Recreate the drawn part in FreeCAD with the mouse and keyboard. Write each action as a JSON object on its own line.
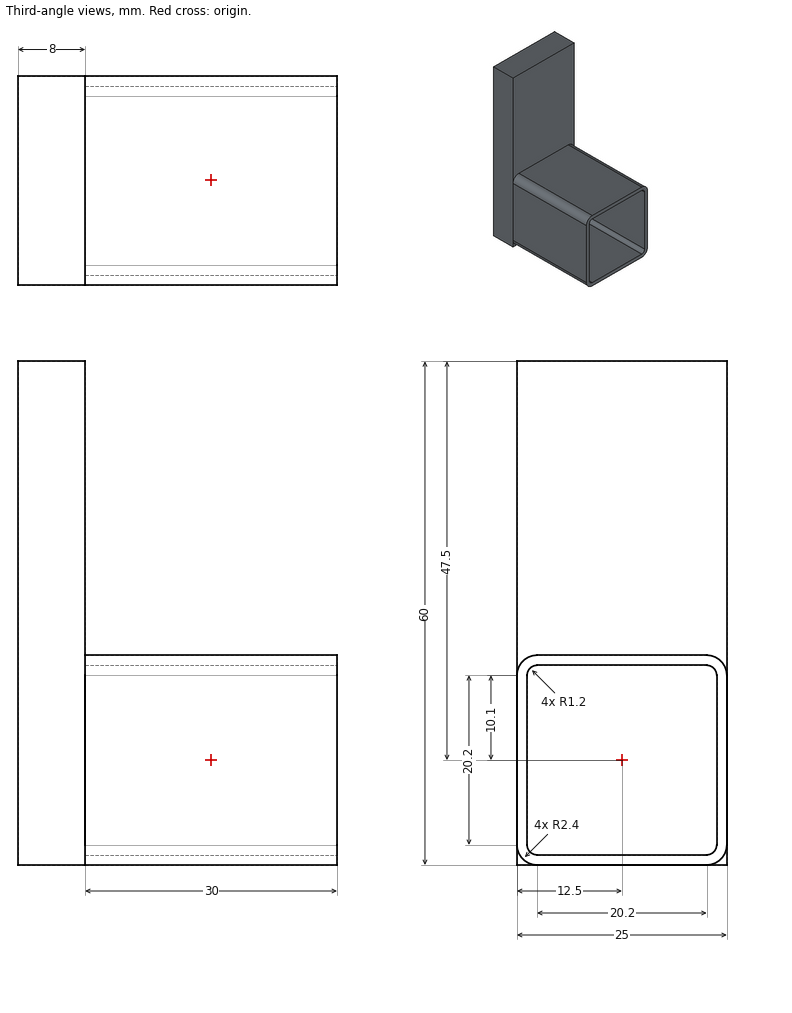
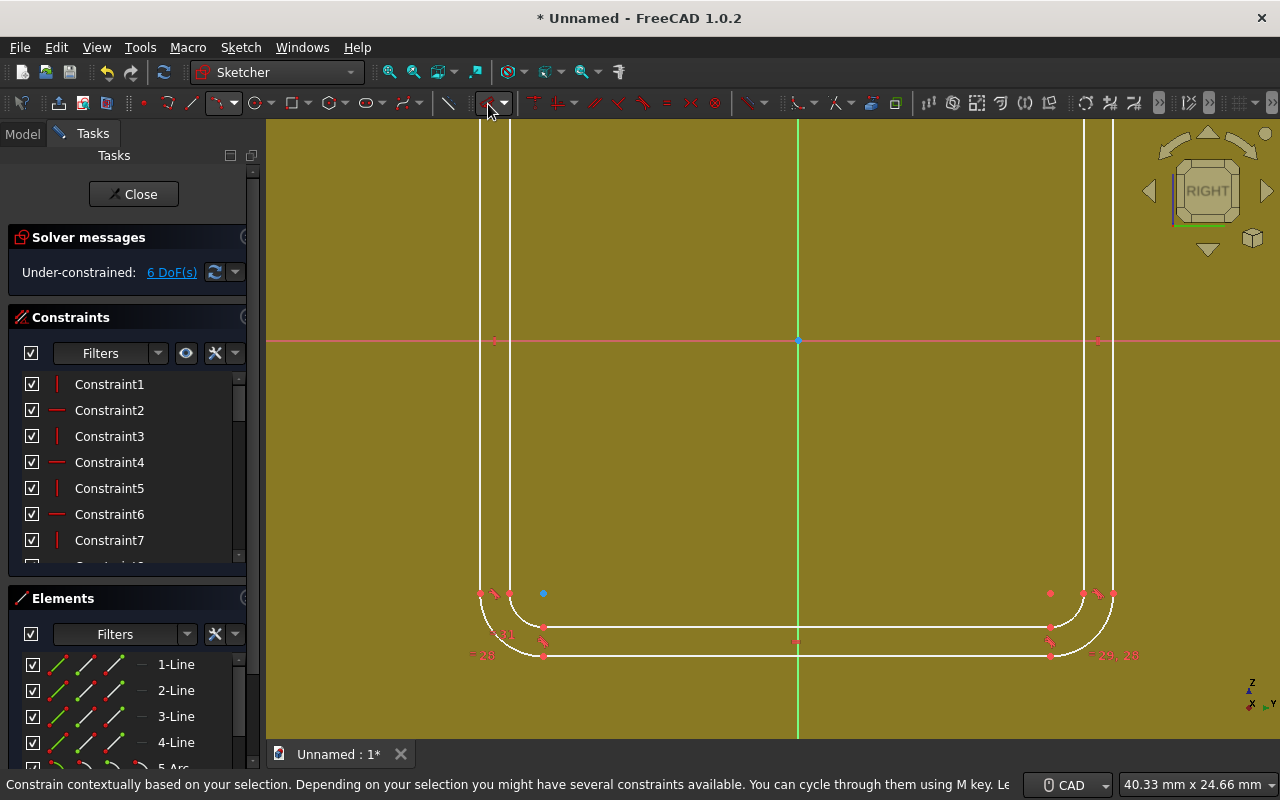
{"action": "left_click", "coordinate": [487, 622]}
{"action": "left_click", "coordinate": [458, 637]}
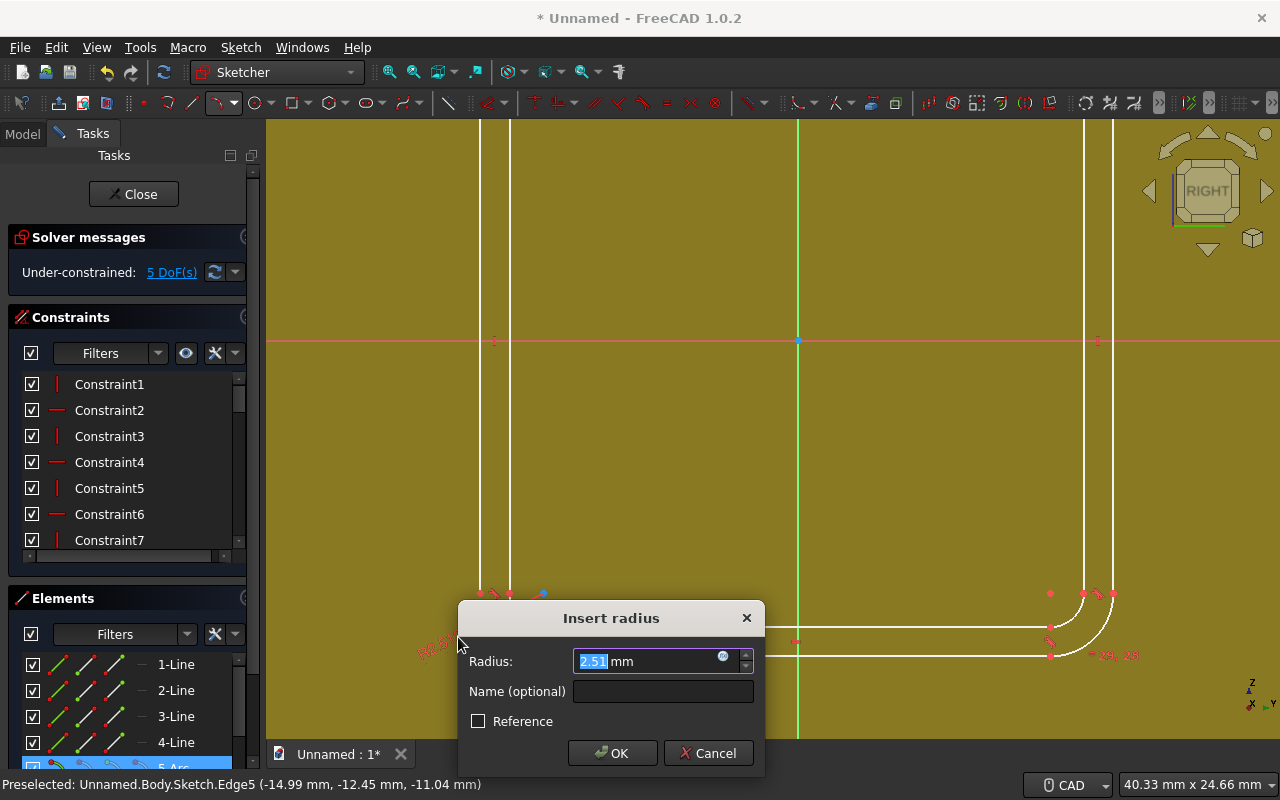
{"action": "type", "text": "2.4"}
{"action": "key", "text": "Return"}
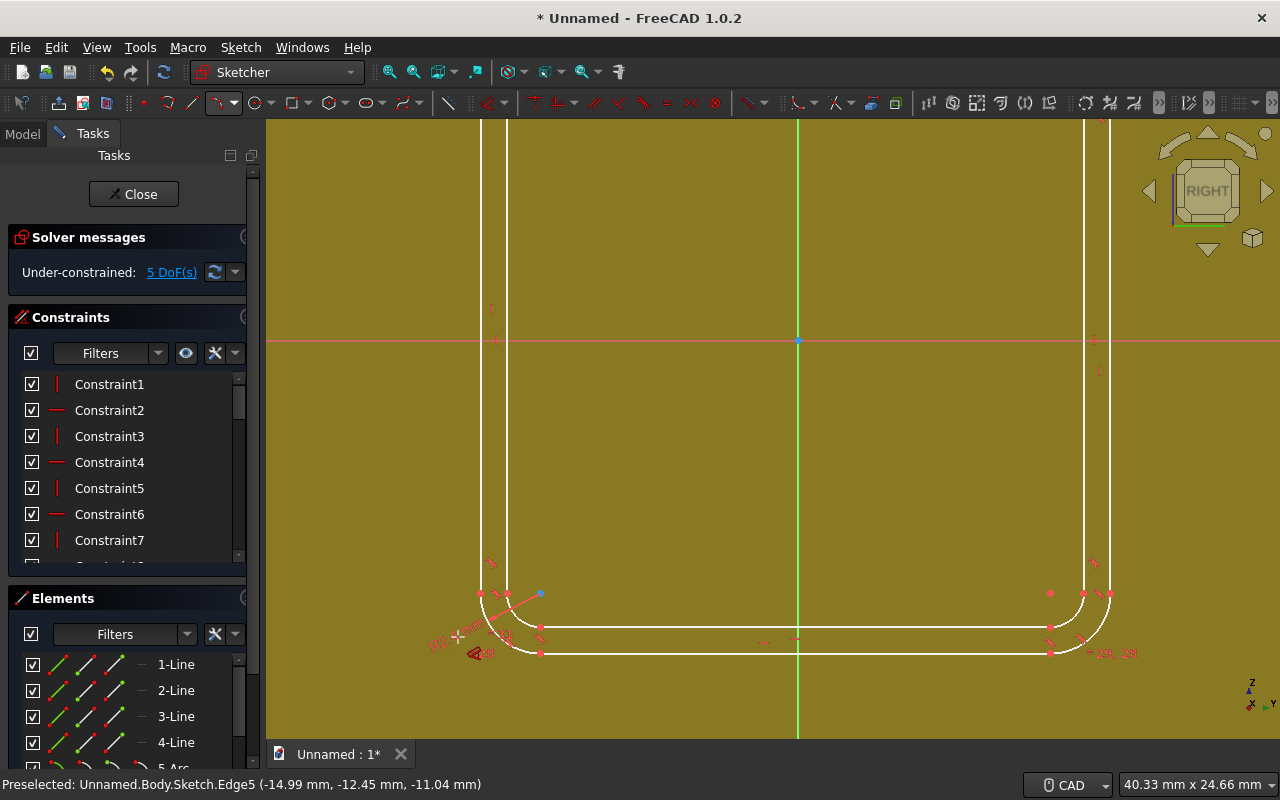
{"action": "scroll", "coordinate": [514, 608], "scroll_direction": "down", "scroll_amount": 2}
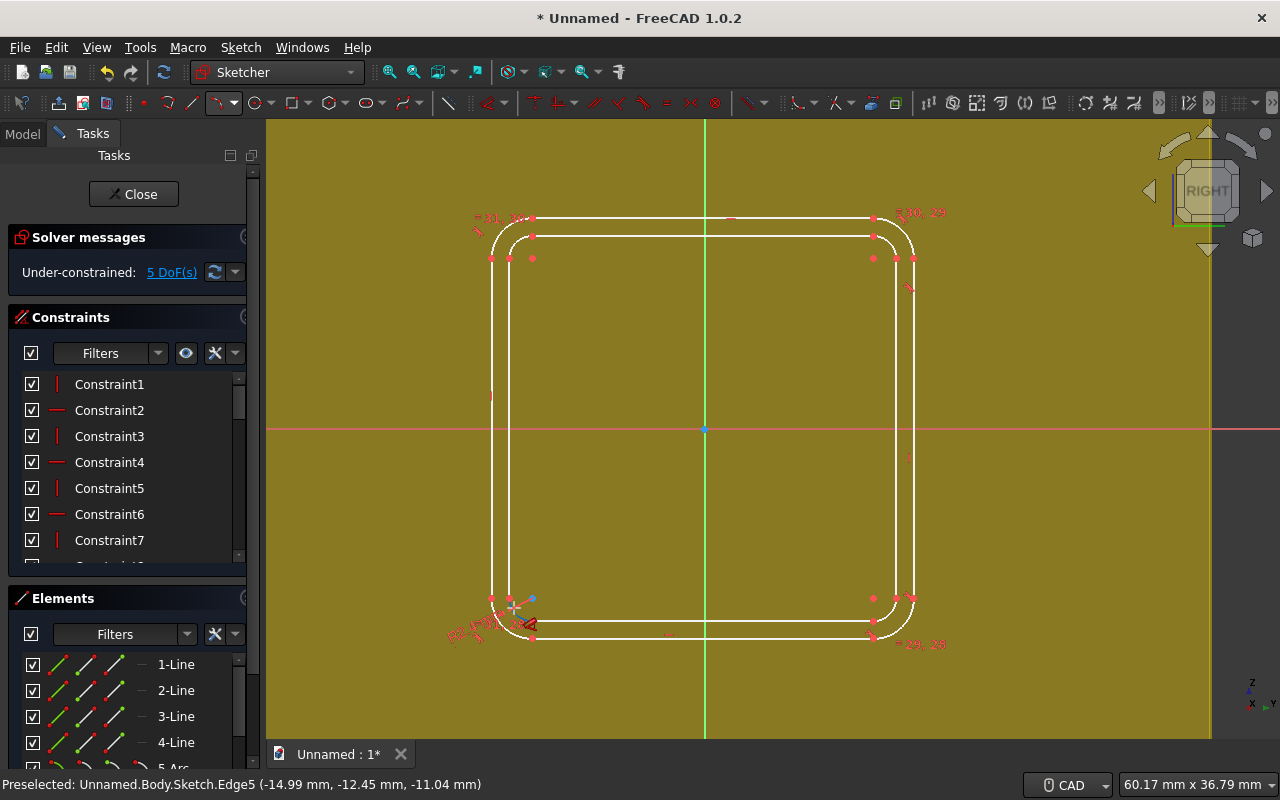
{"action": "scroll", "coordinate": [522, 239], "scroll_direction": "up", "scroll_amount": 4}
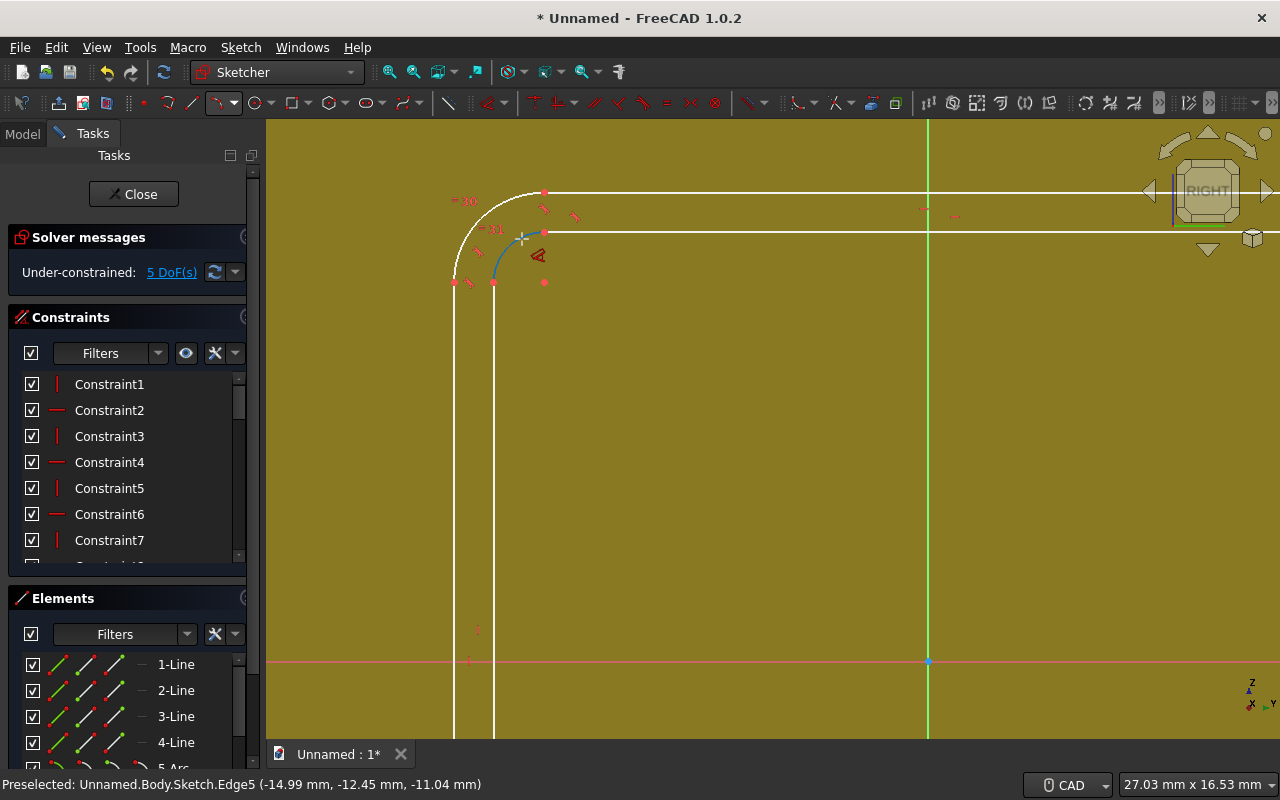
{"action": "left_click", "coordinate": [521, 238]}
{"action": "left_click", "coordinate": [585, 211]}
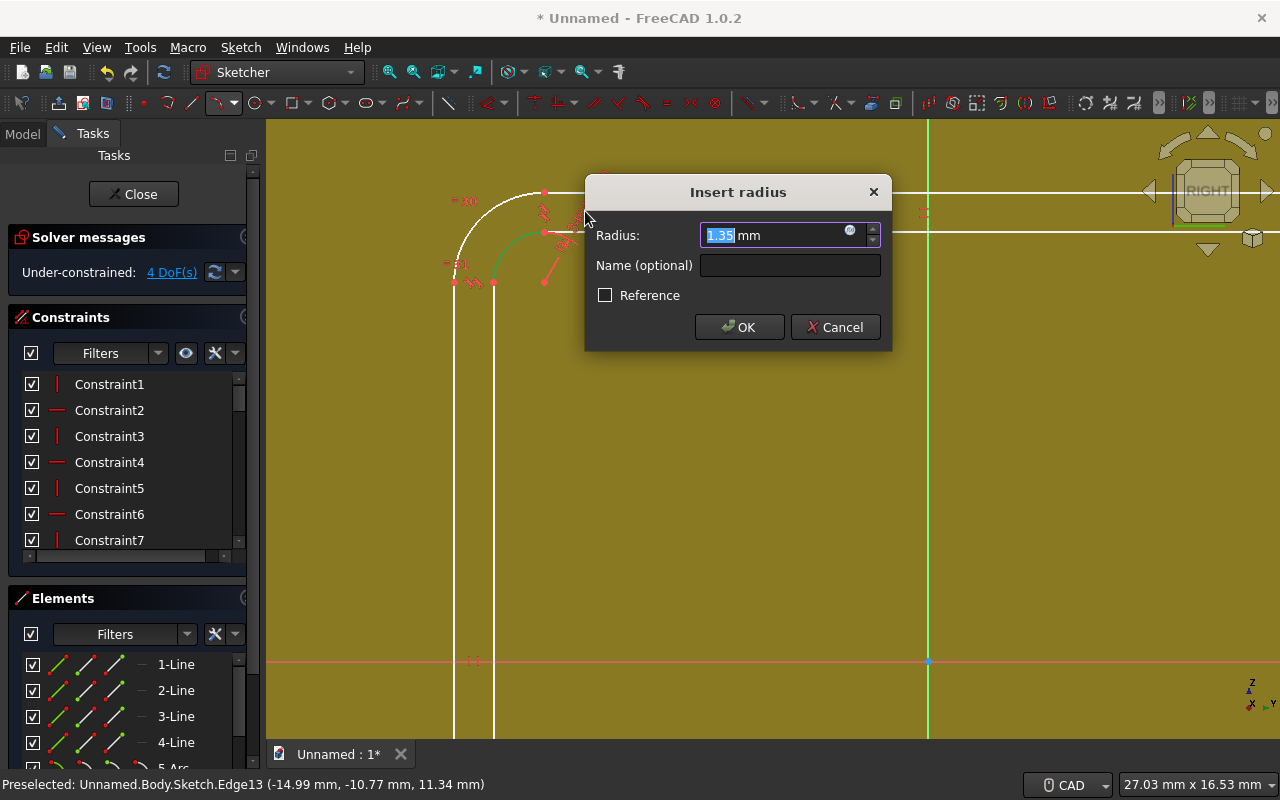
{"action": "type", "text": "1.2"}
{"action": "key", "text": "Return"}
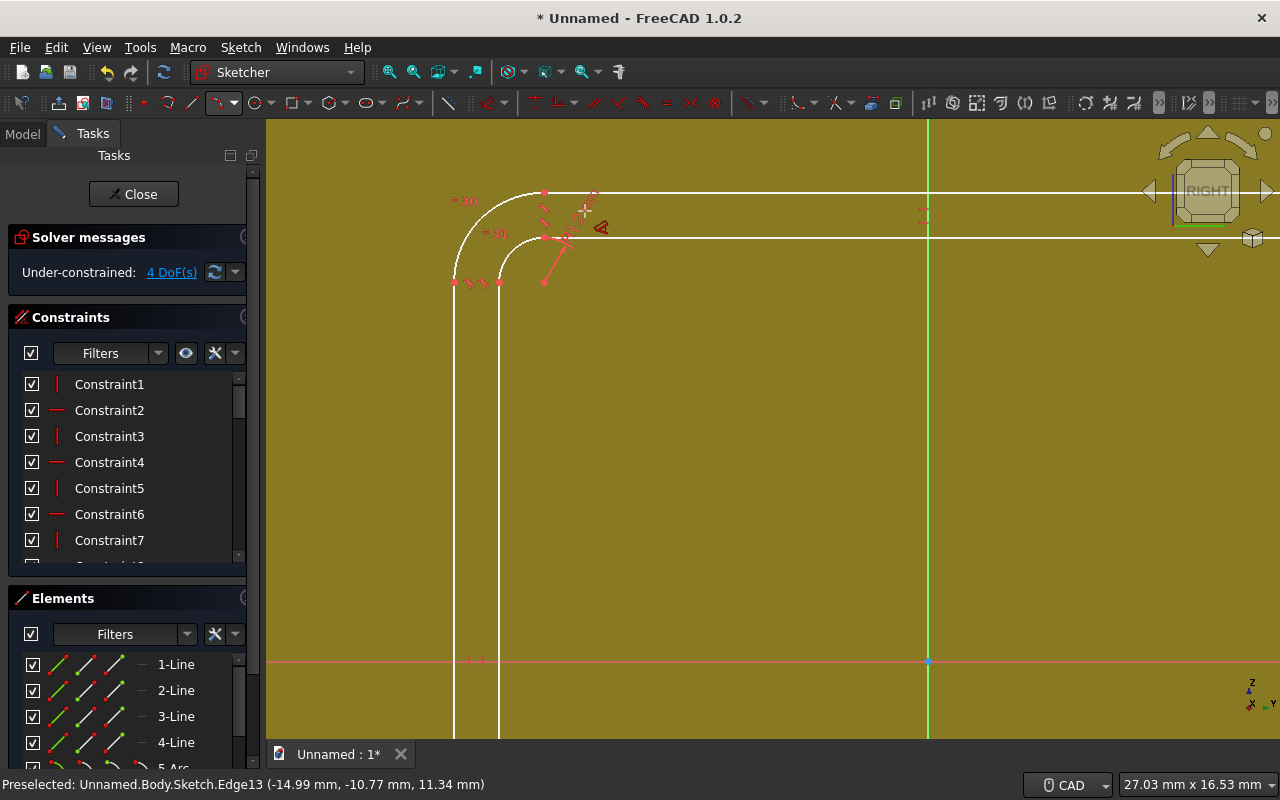
{"action": "left_click", "coordinate": [454, 510]}
{"action": "left_click", "coordinate": [420, 497]}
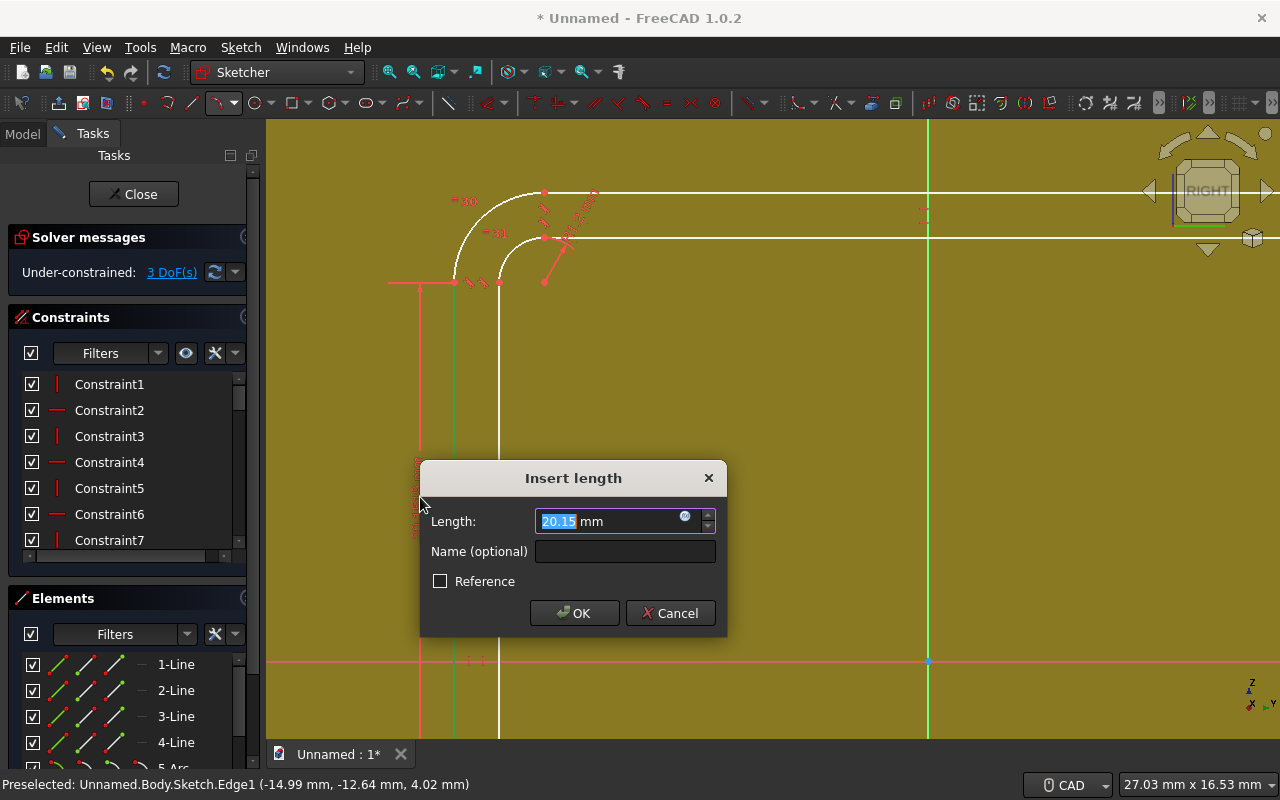
{"action": "type", "text": "20.2"}
{"action": "key", "text": "Return"}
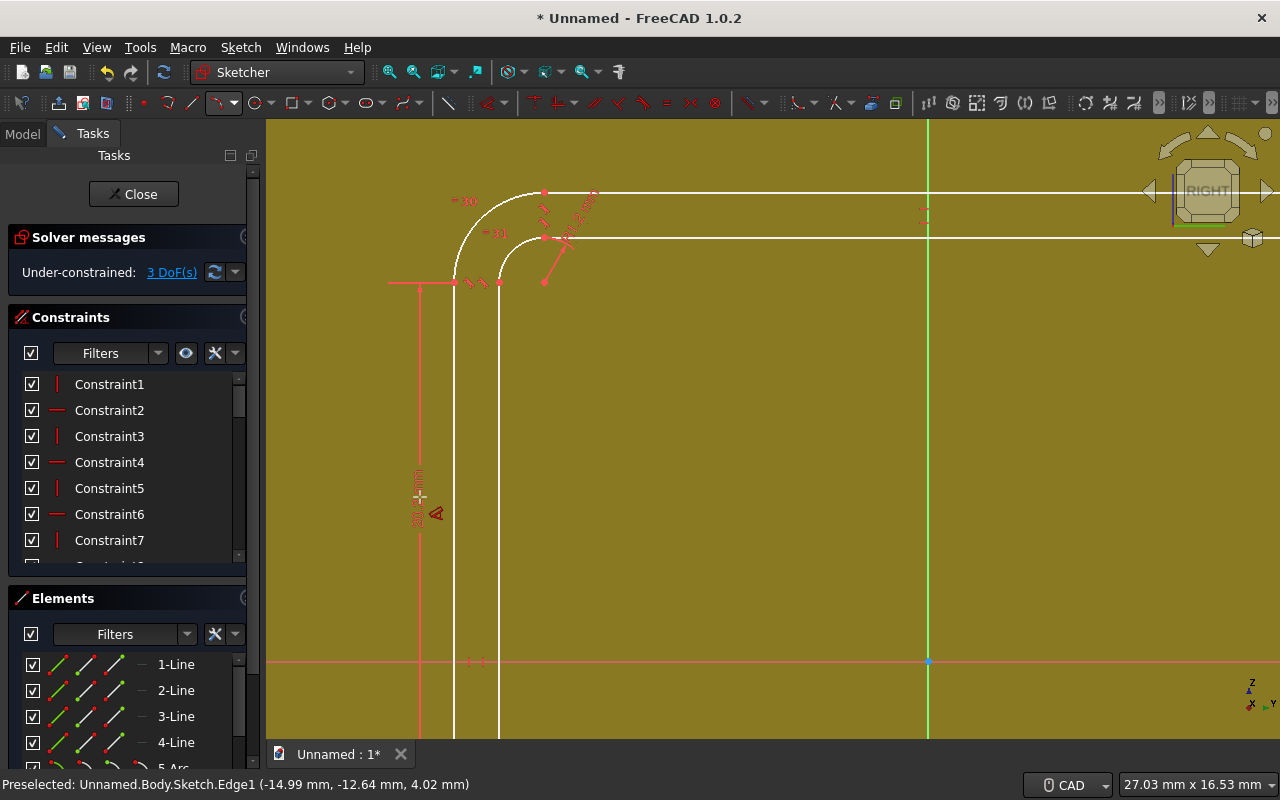
{"action": "scroll", "coordinate": [522, 239], "scroll_direction": "down", "scroll_amount": 4}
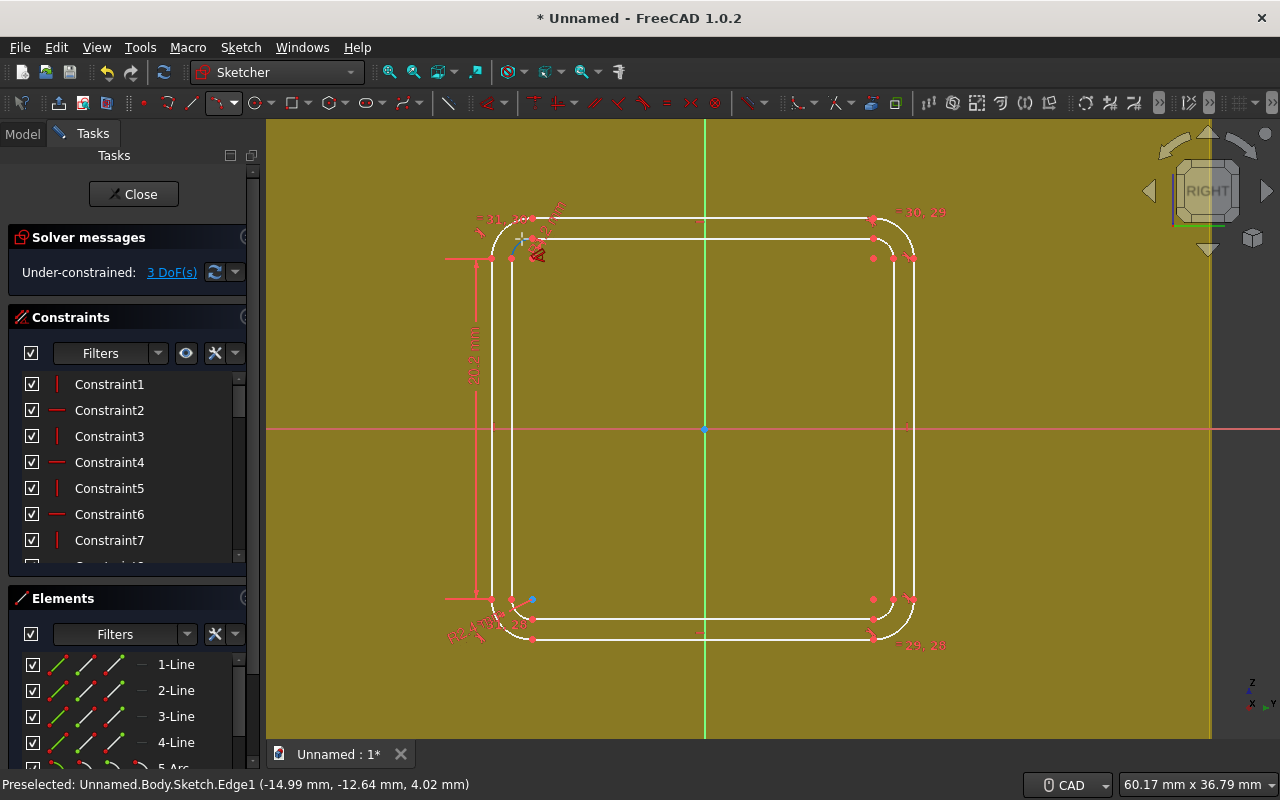
{"action": "left_click", "coordinate": [635, 640]}
{"action": "left_click", "coordinate": [624, 674]}